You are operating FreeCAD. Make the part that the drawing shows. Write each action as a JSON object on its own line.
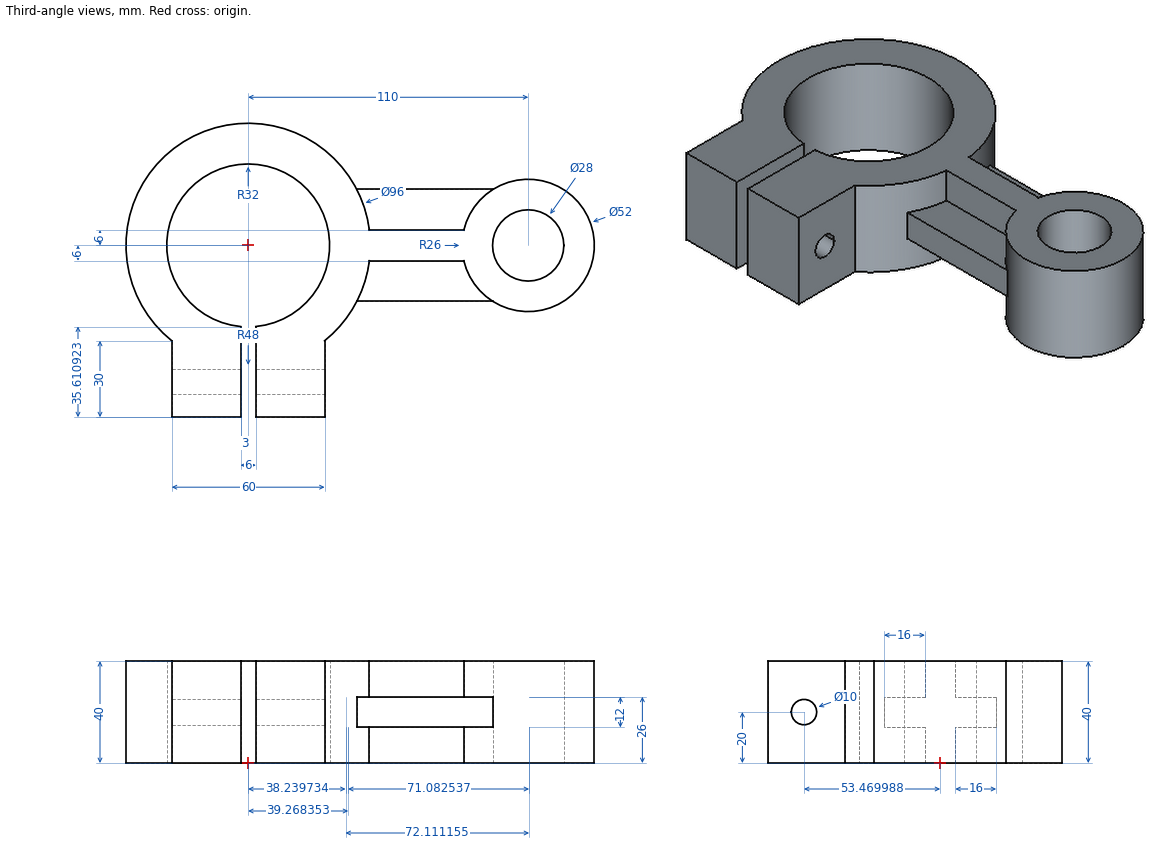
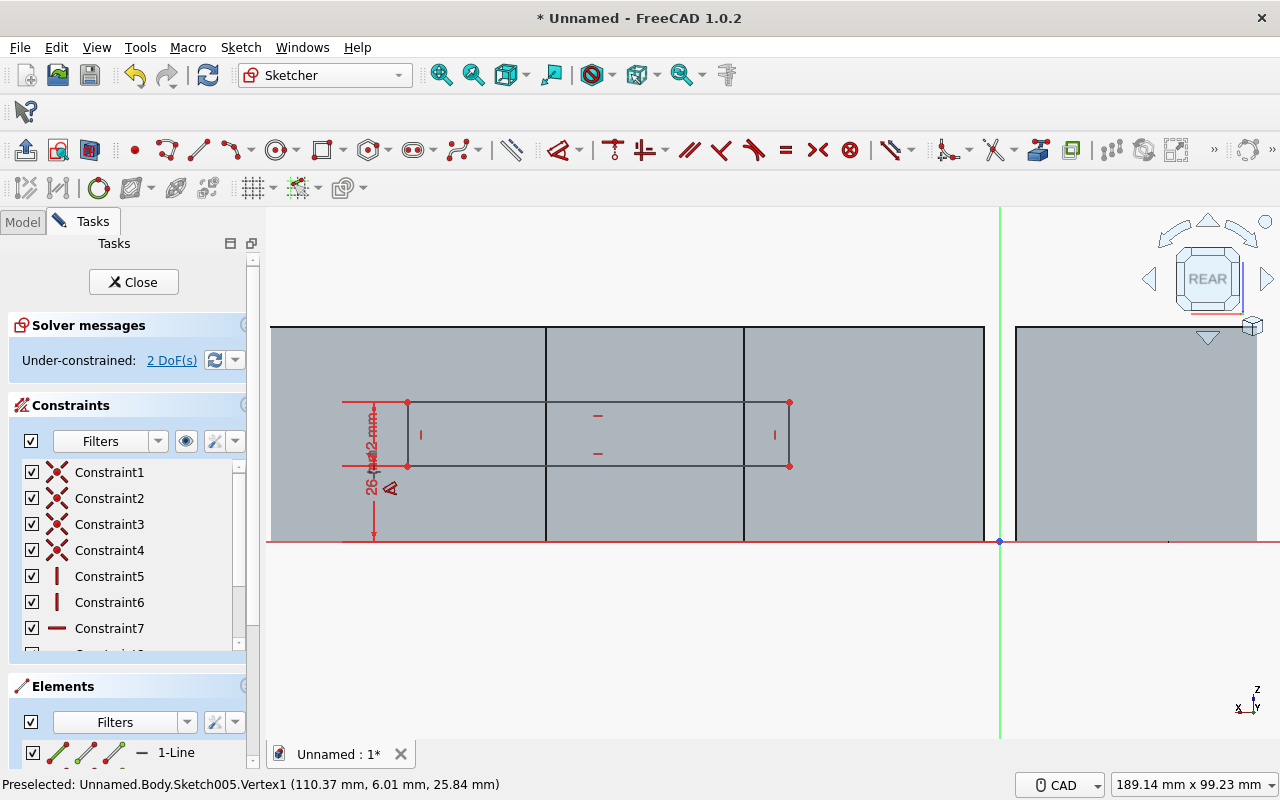
{"action": "left_click", "coordinate": [522, 466]}
{"action": "left_click", "coordinate": [598, 432]}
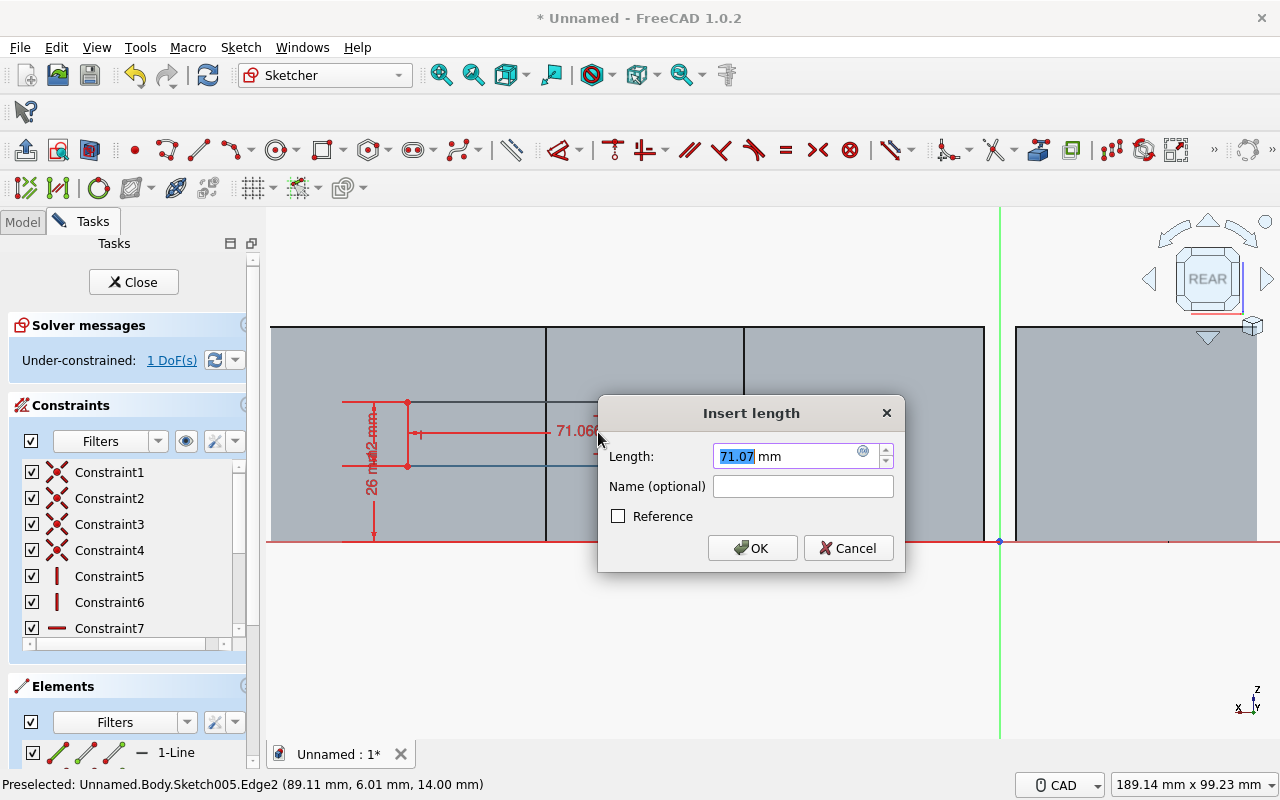
{"action": "type", "text": "71.082537"}
{"action": "key", "text": "Return"}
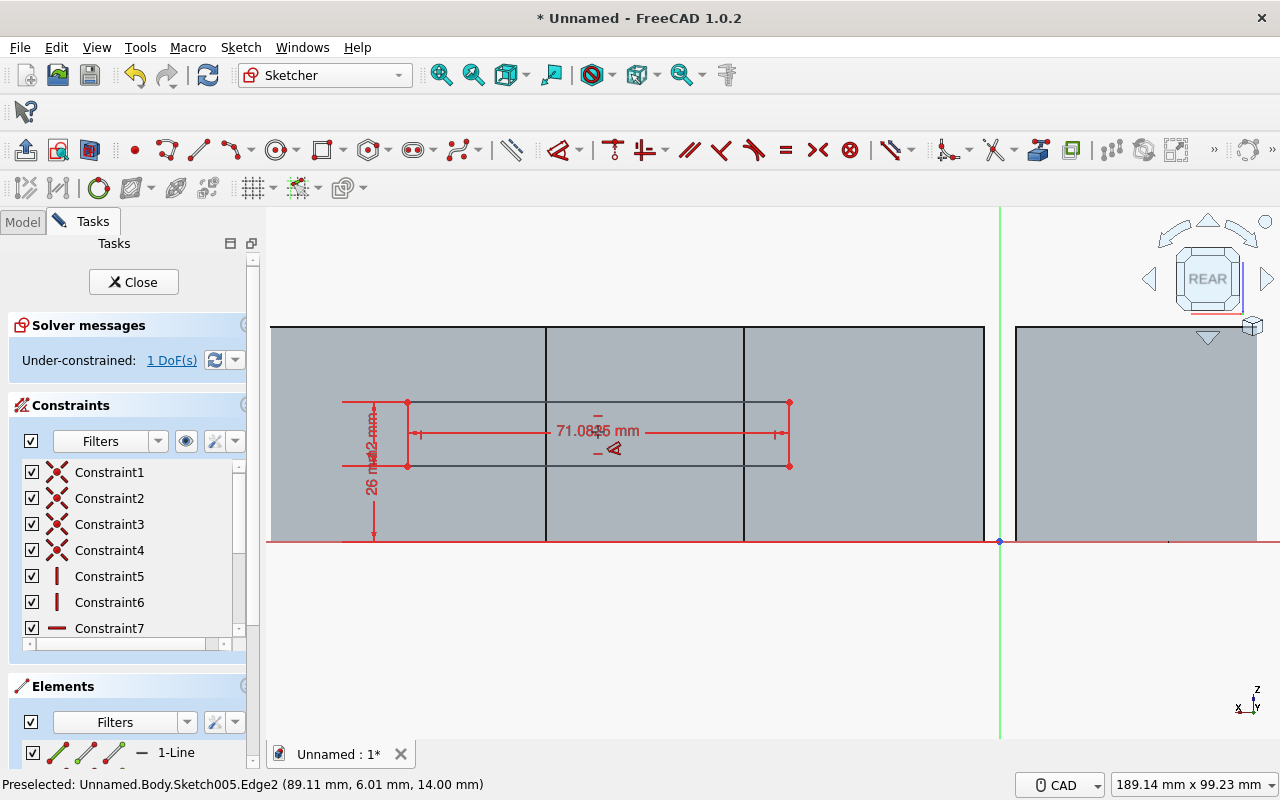
{"action": "left_click", "coordinate": [789, 466]}
{"action": "left_click", "coordinate": [894, 576]}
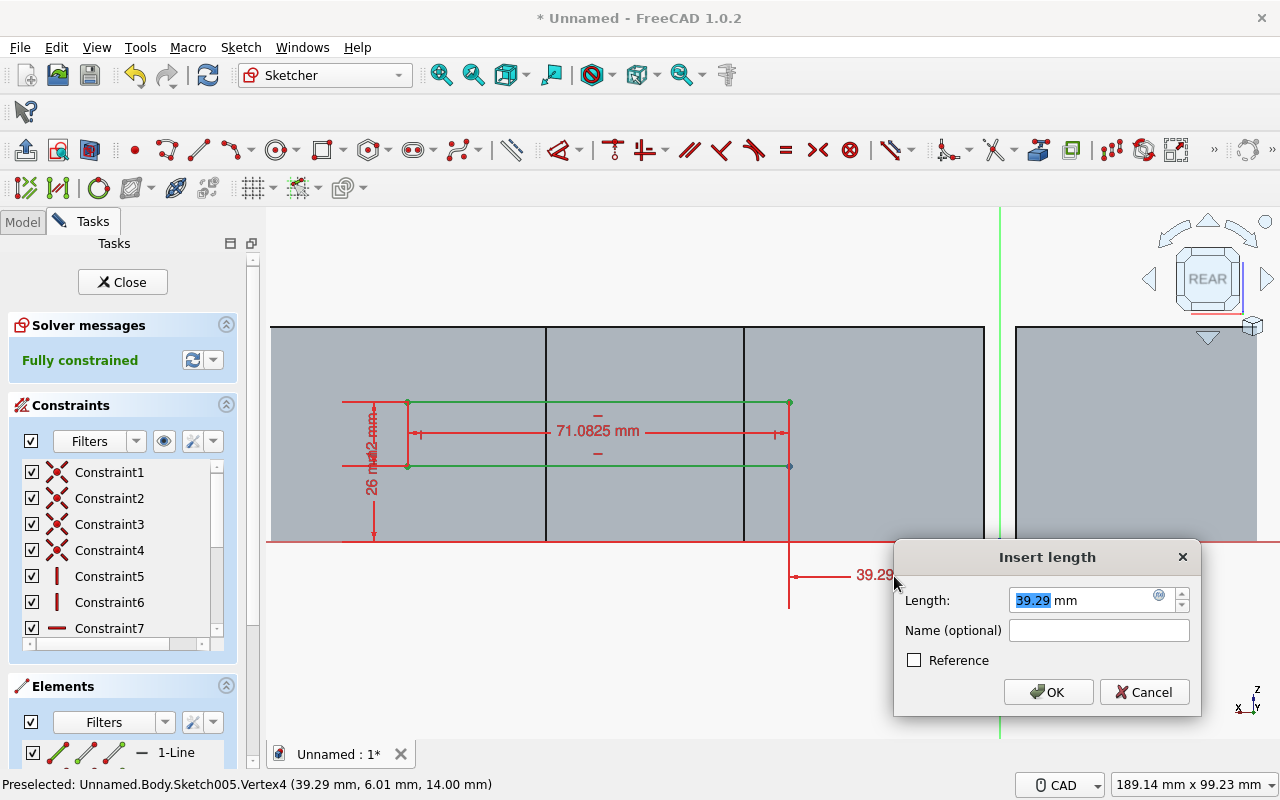
{"action": "type", "text": "39.268353"}
{"action": "key", "text": "Return"}
{"action": "key", "text": "Escape"}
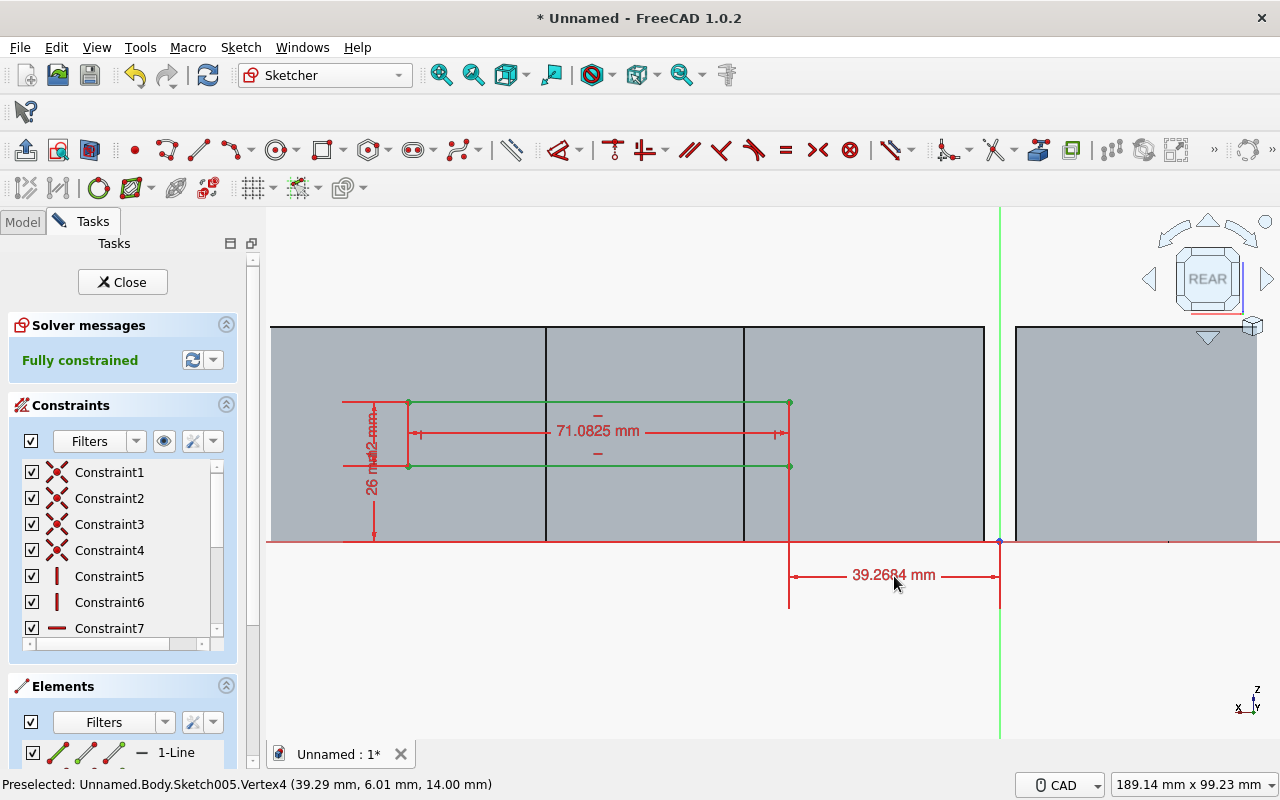
{"action": "left_click", "coordinate": [123, 282]}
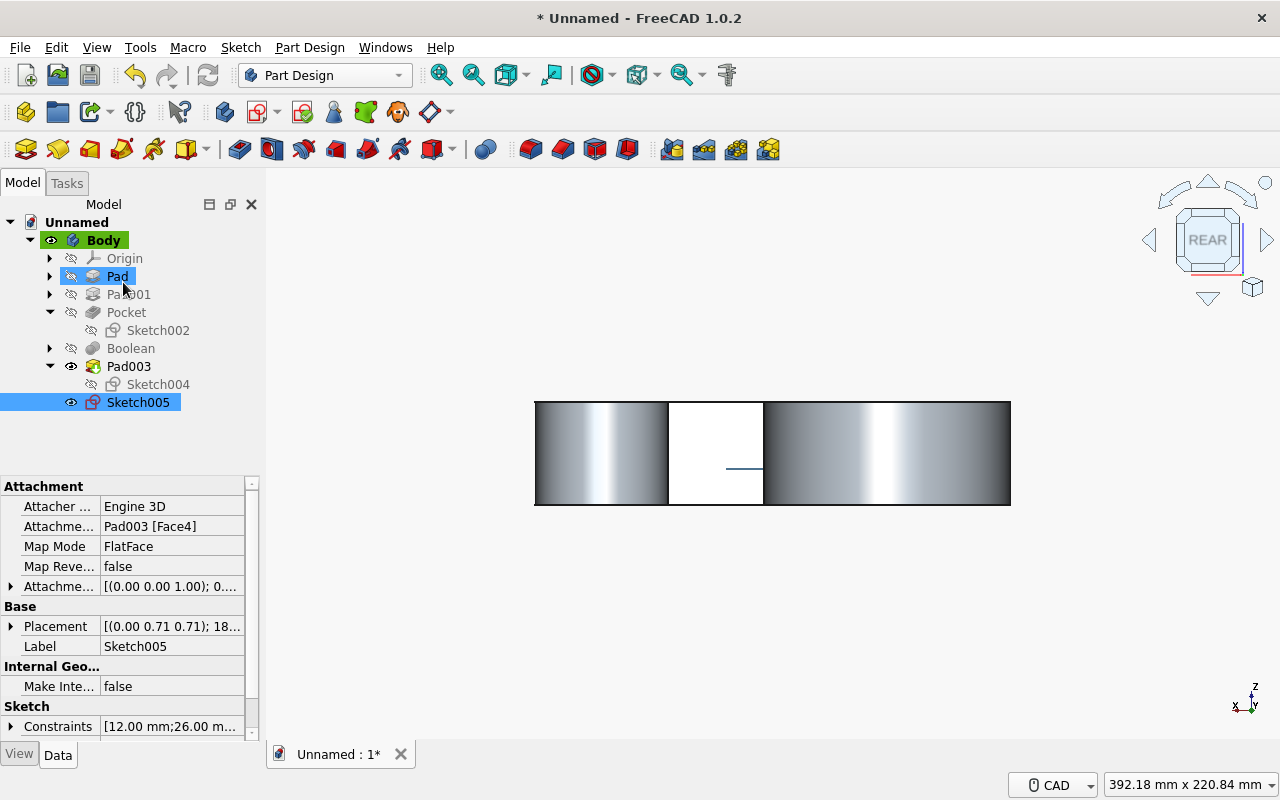
{"action": "left_click", "coordinate": [26, 150]}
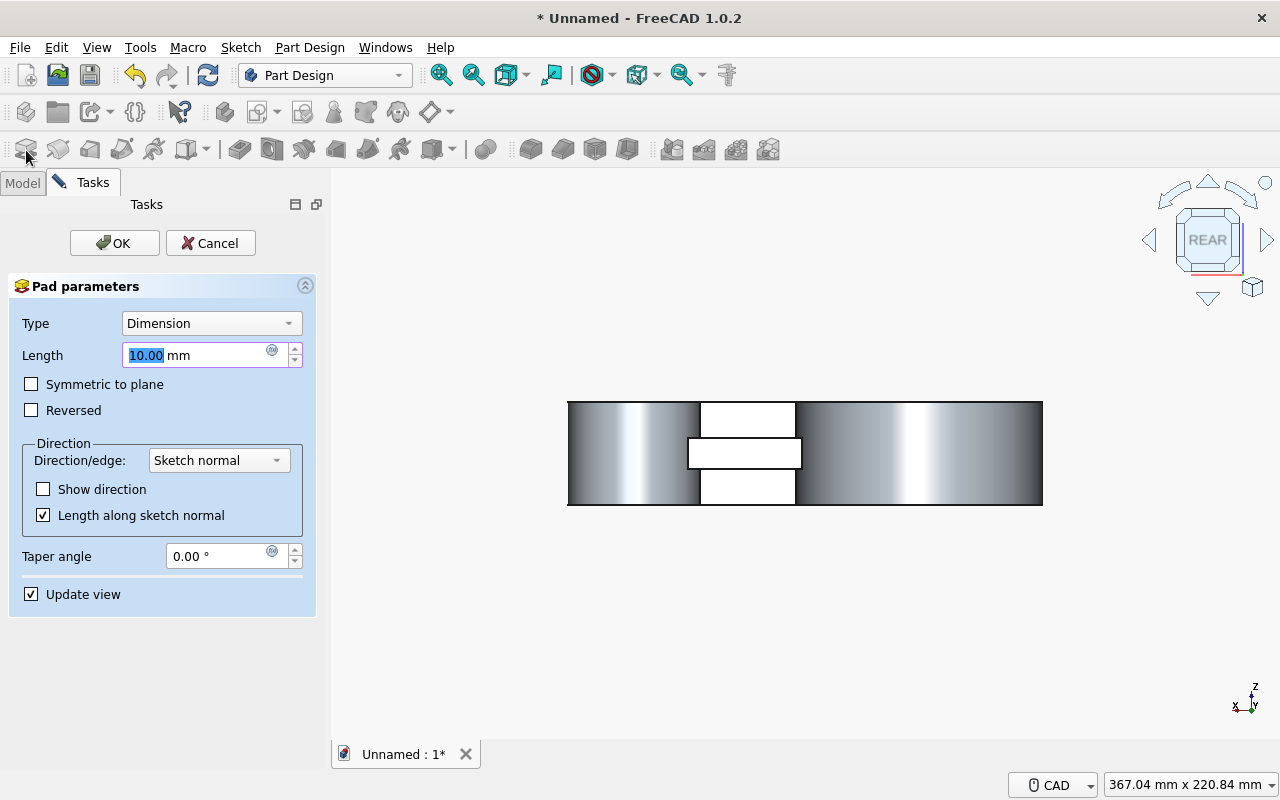
{"action": "type", "text": "16"}
{"action": "key", "text": "Tab"}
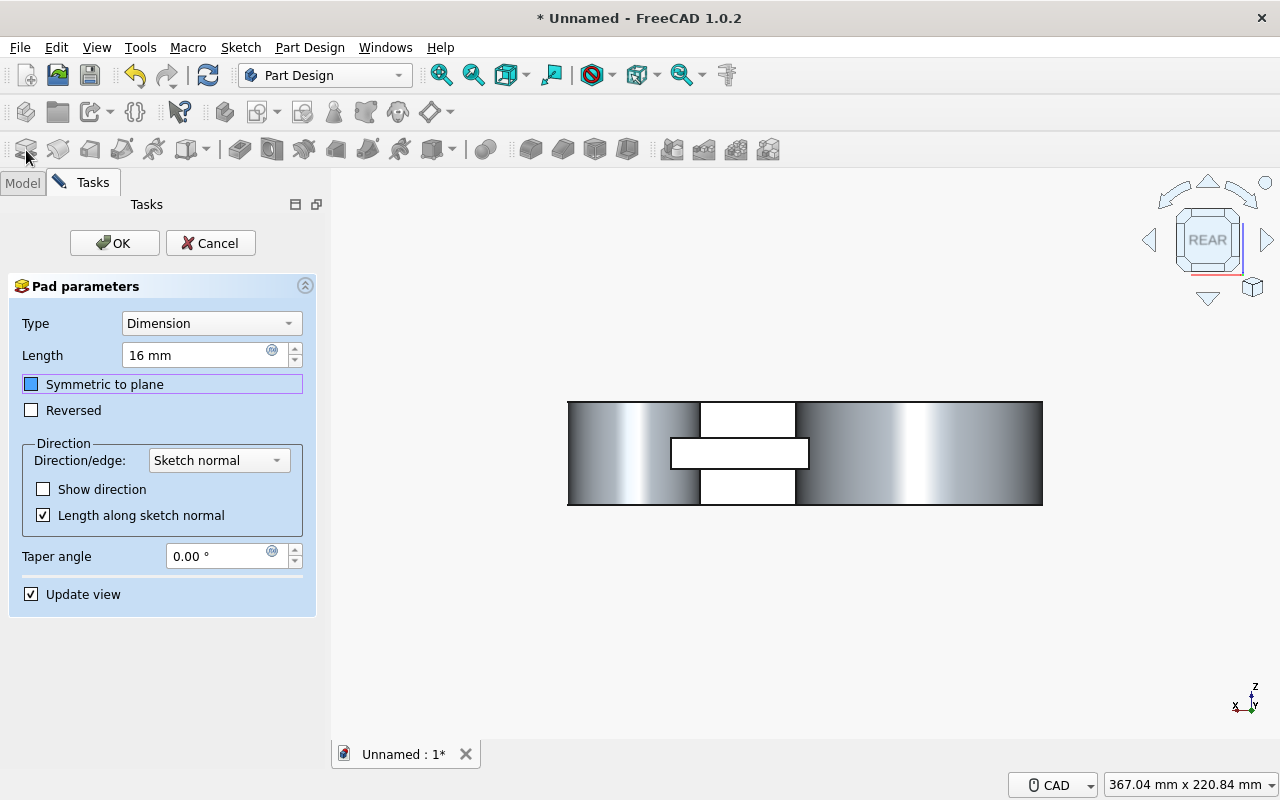
{"action": "left_click", "coordinate": [115, 243]}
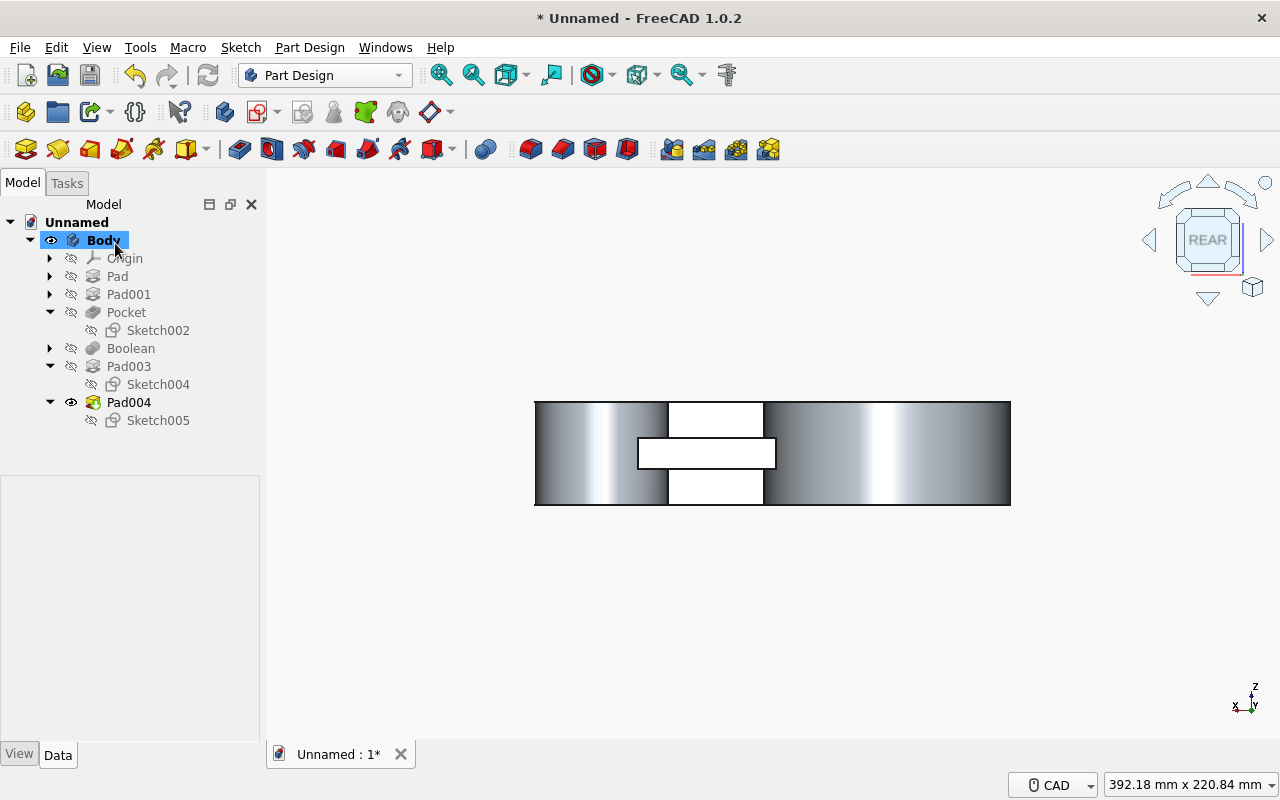
{"action": "key", "text": "0"}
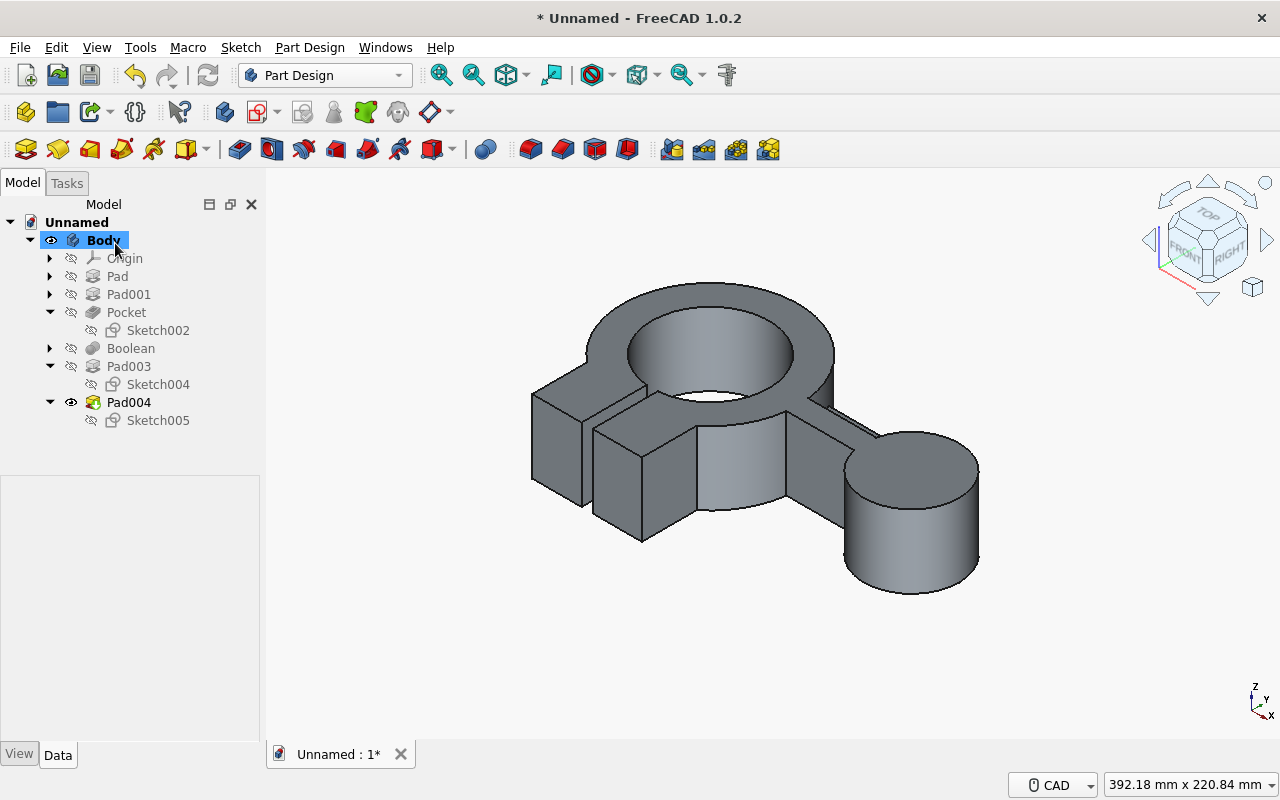
{"action": "left_click", "coordinate": [820, 472]}